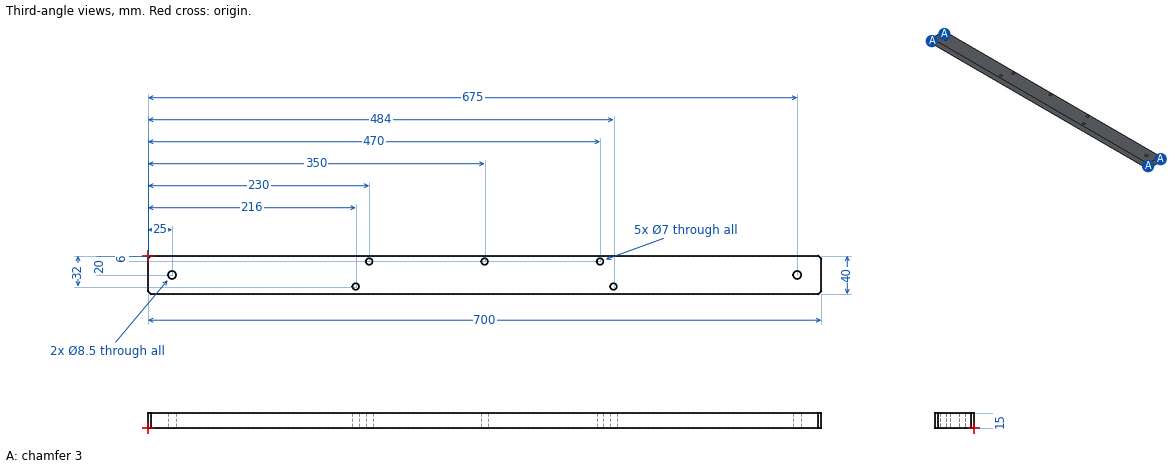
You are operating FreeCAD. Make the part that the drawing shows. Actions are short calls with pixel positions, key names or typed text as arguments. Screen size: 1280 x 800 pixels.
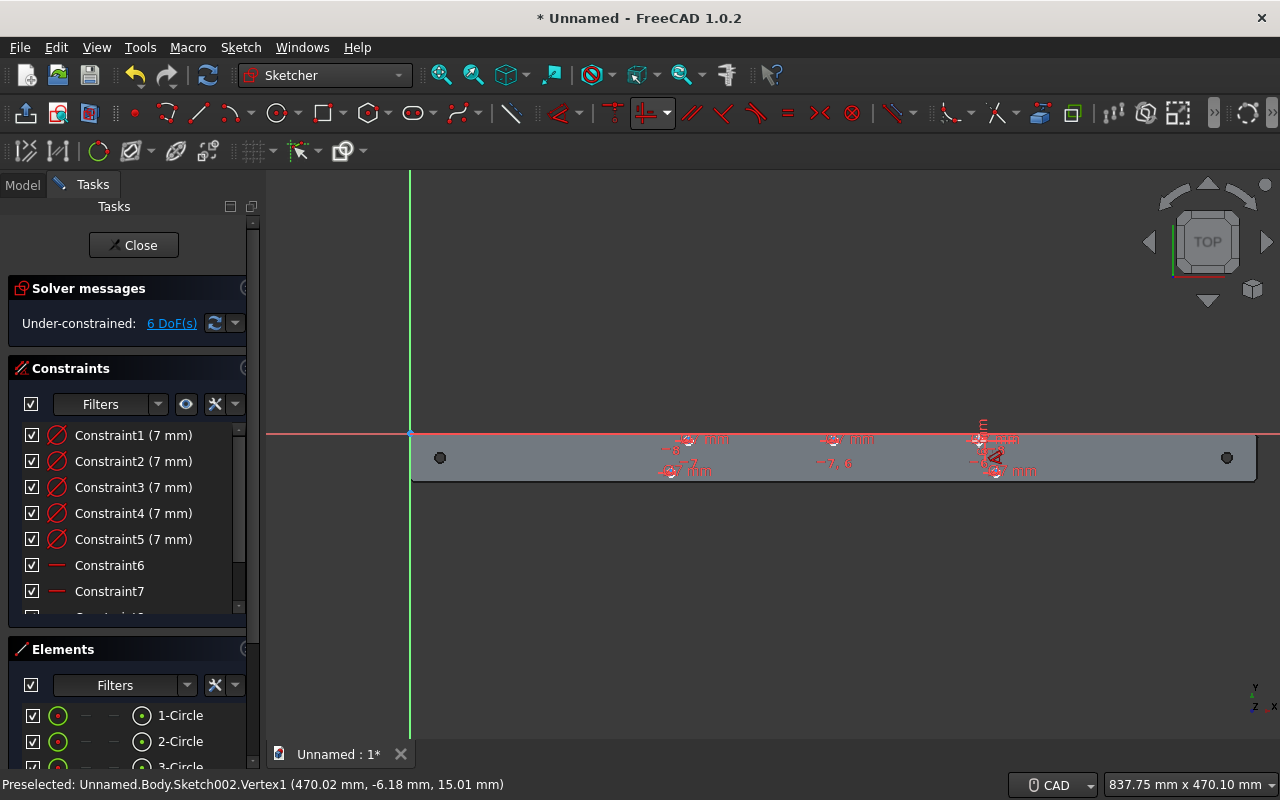
click(671, 473)
click(376, 453)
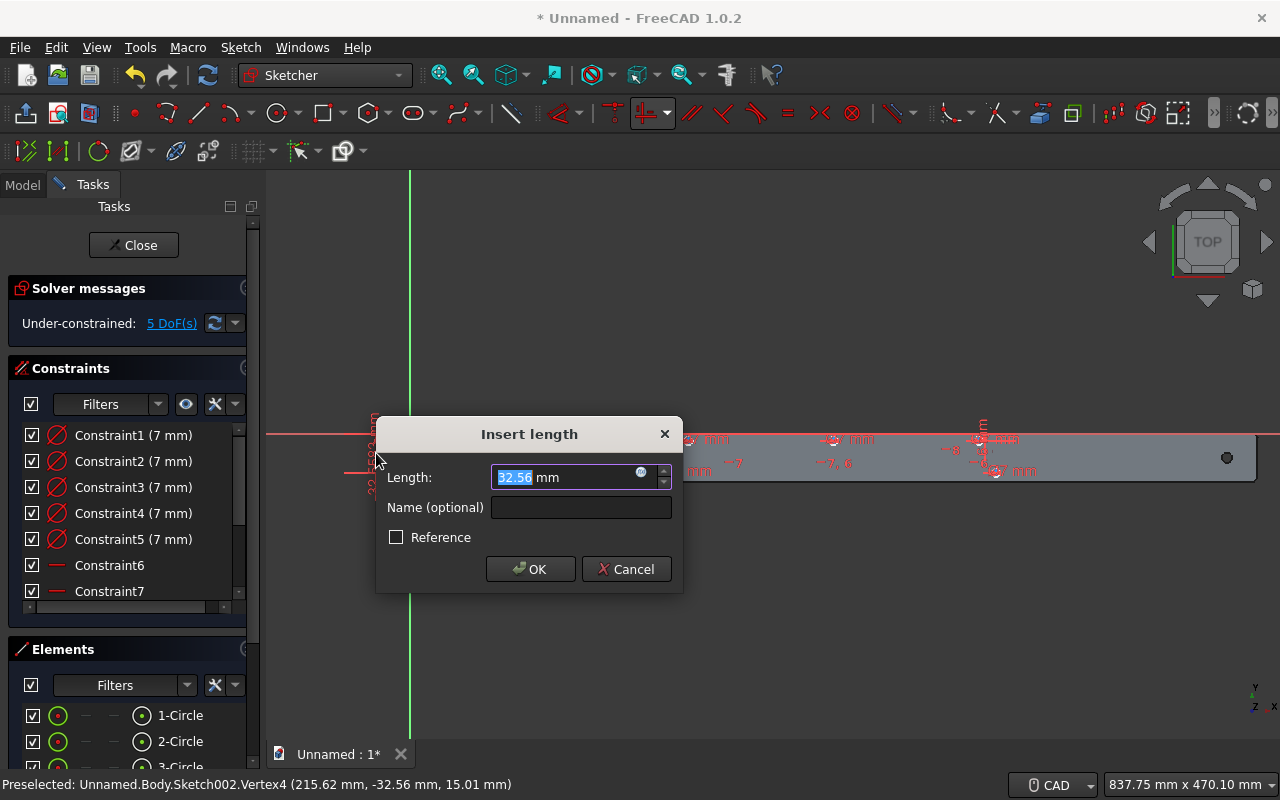
text(32)
key(Return)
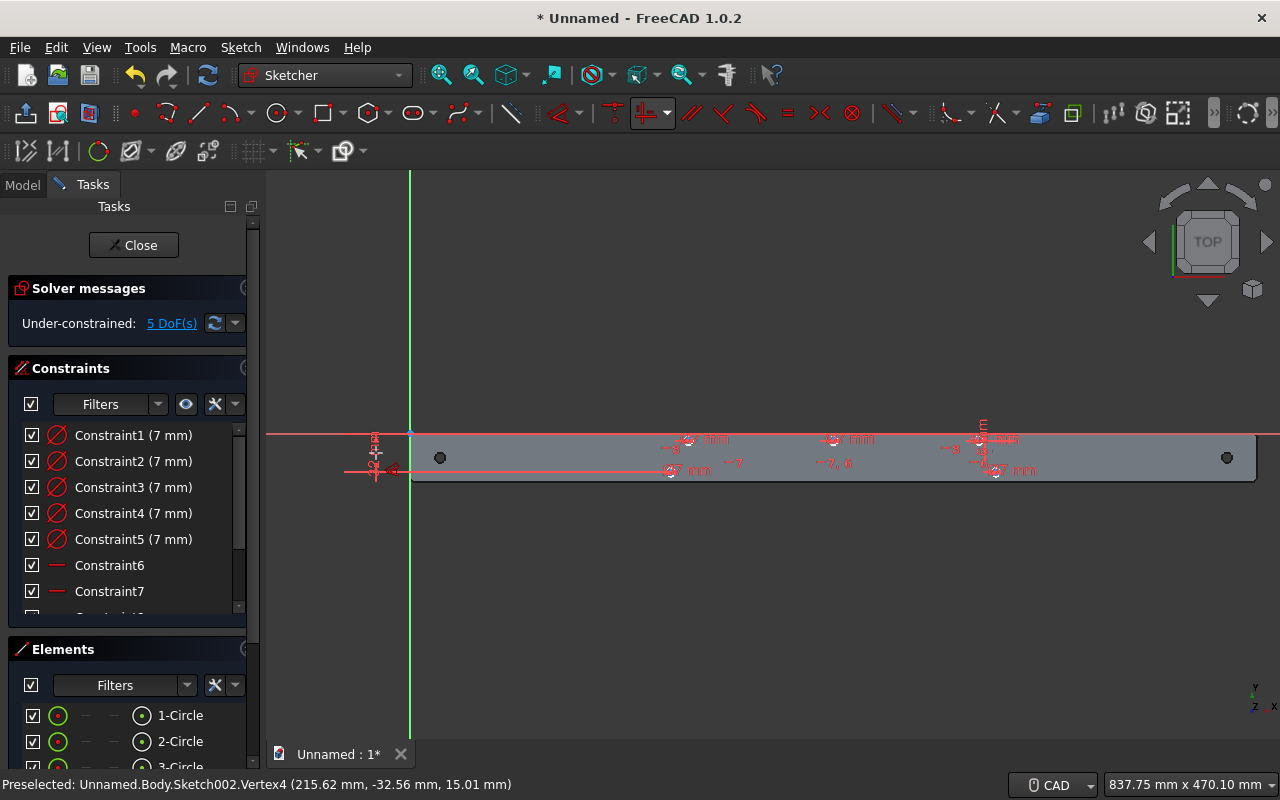
click(979, 441)
click(694, 400)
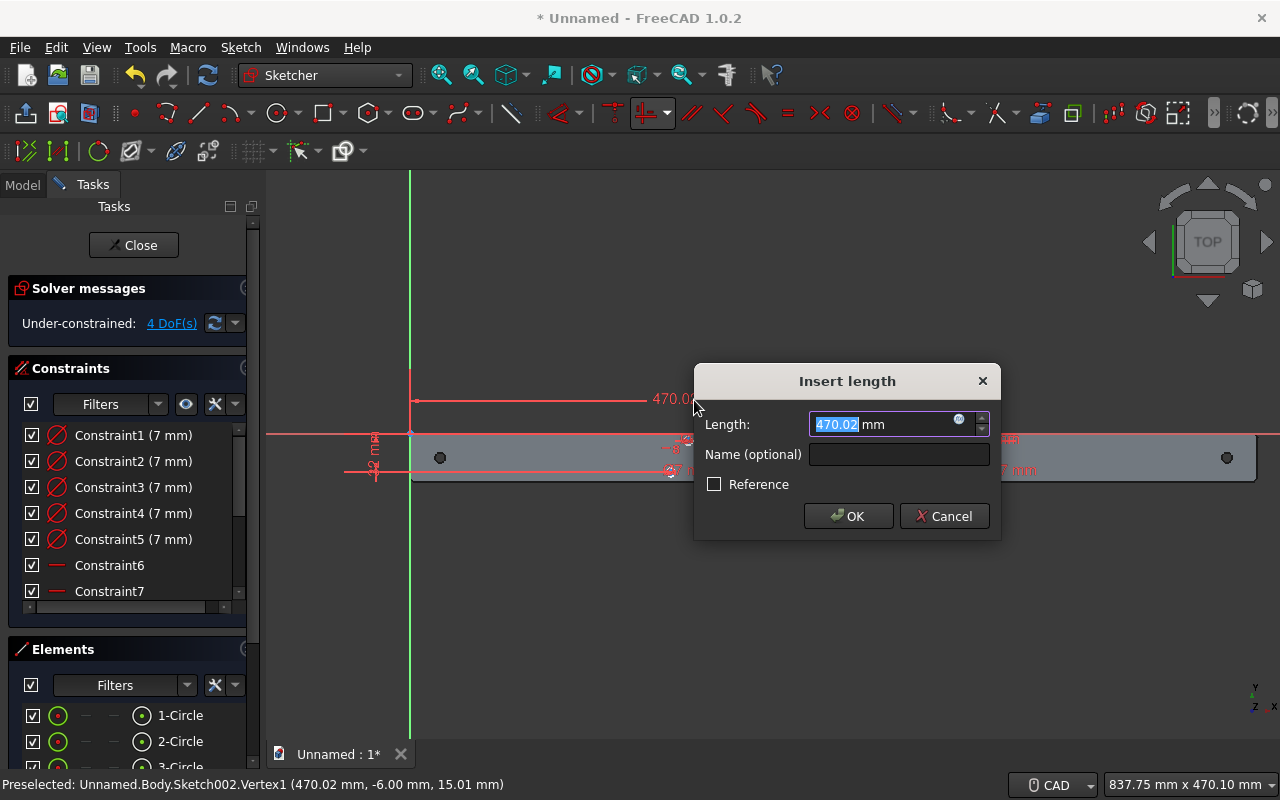
text(470)
key(Return)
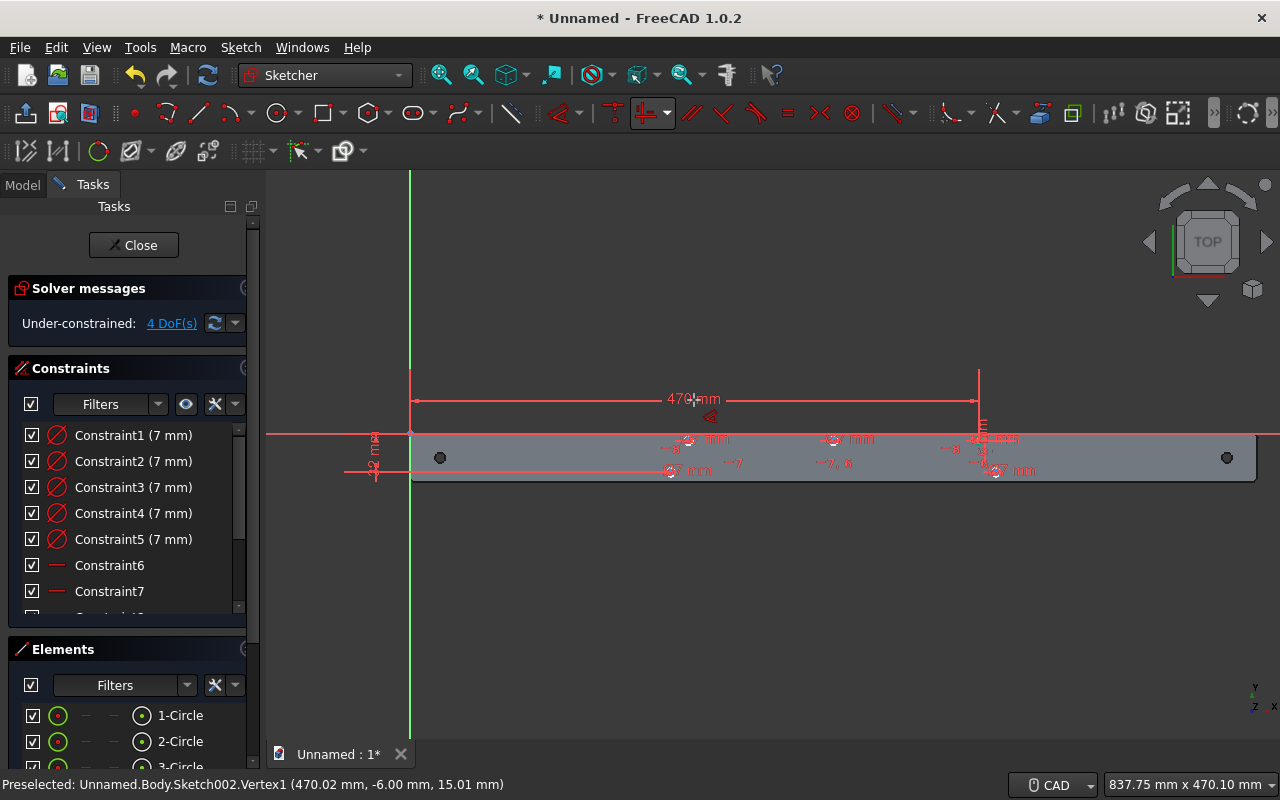
click(834, 441)
click(622, 400)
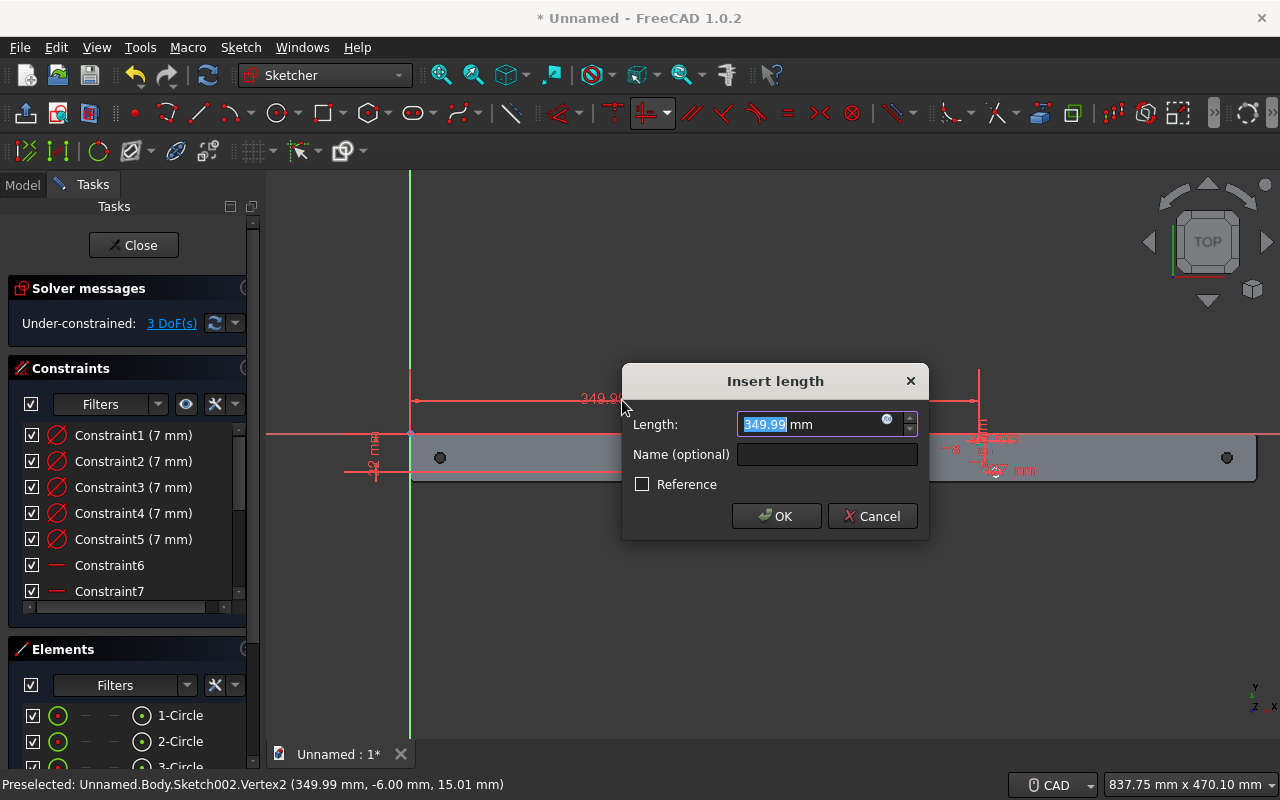
text(350)
key(Return)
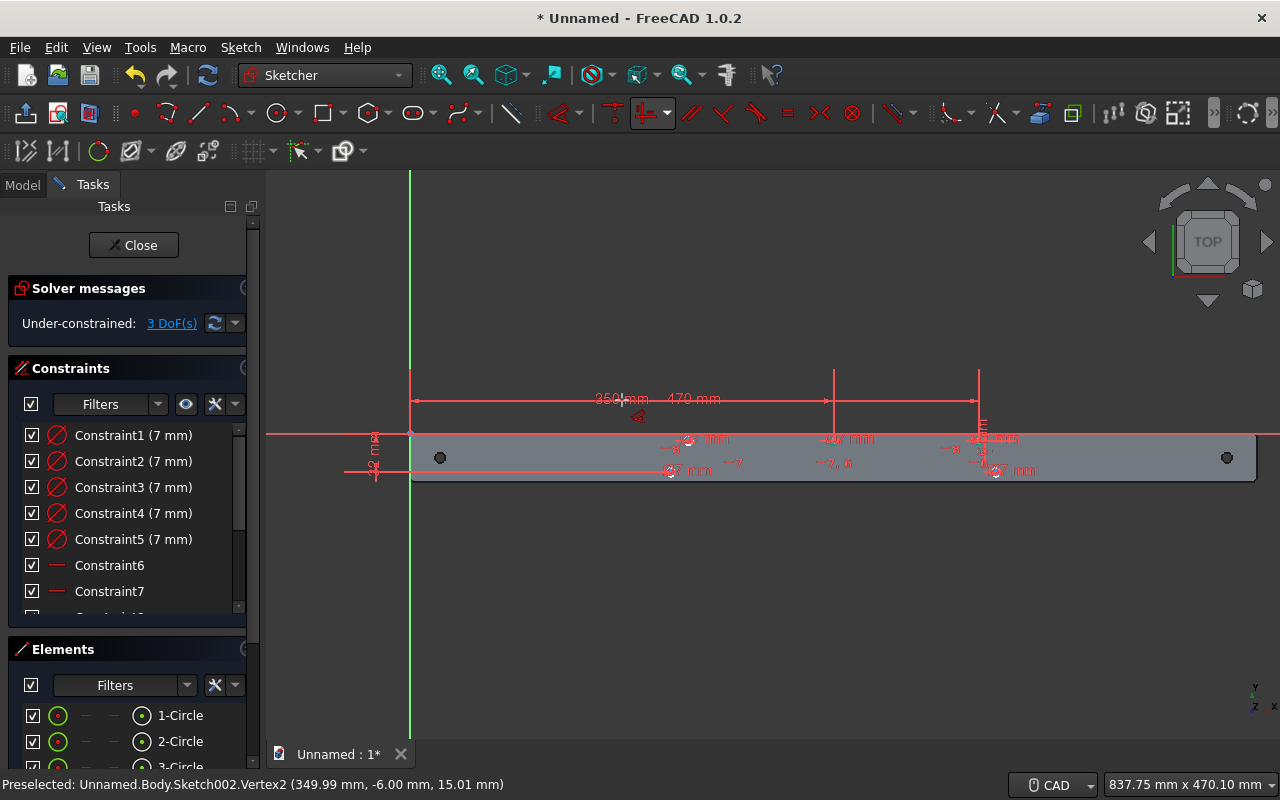
click(688, 441)
click(549, 400)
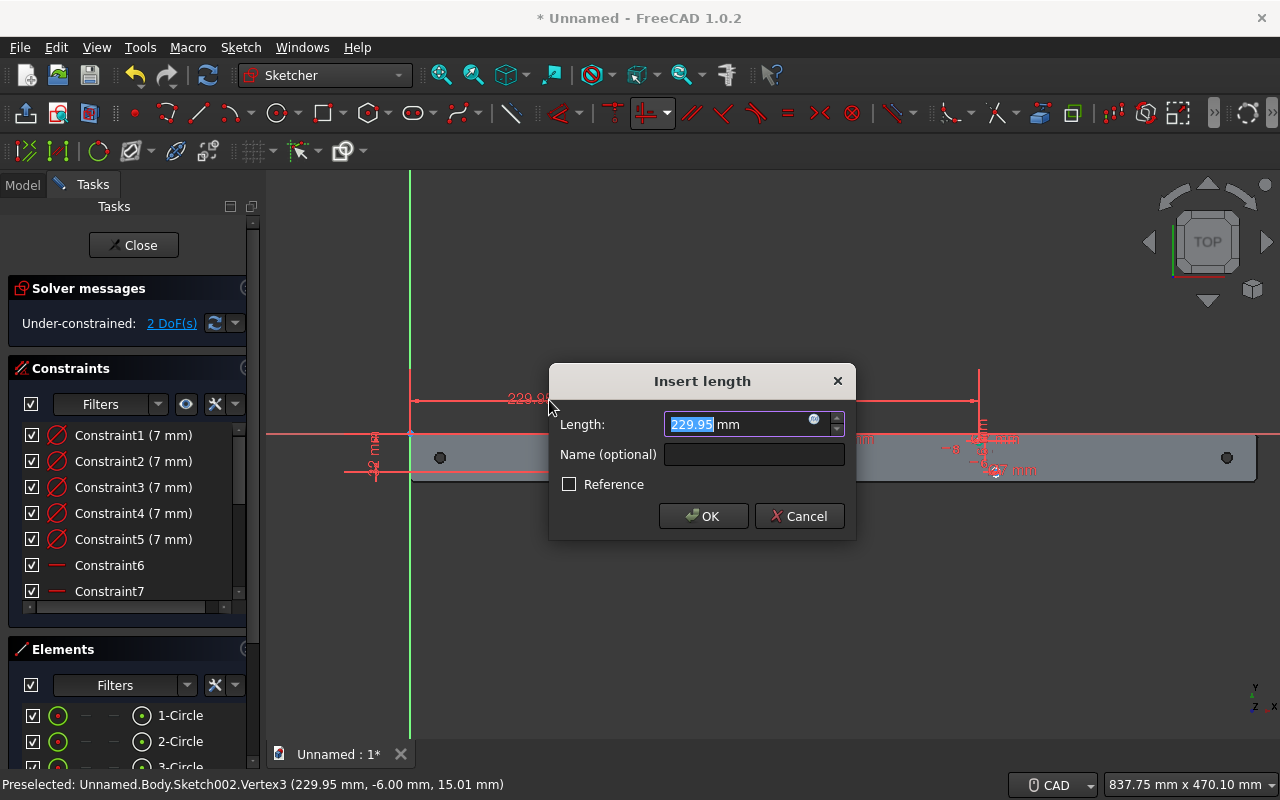
text(230)
key(Return)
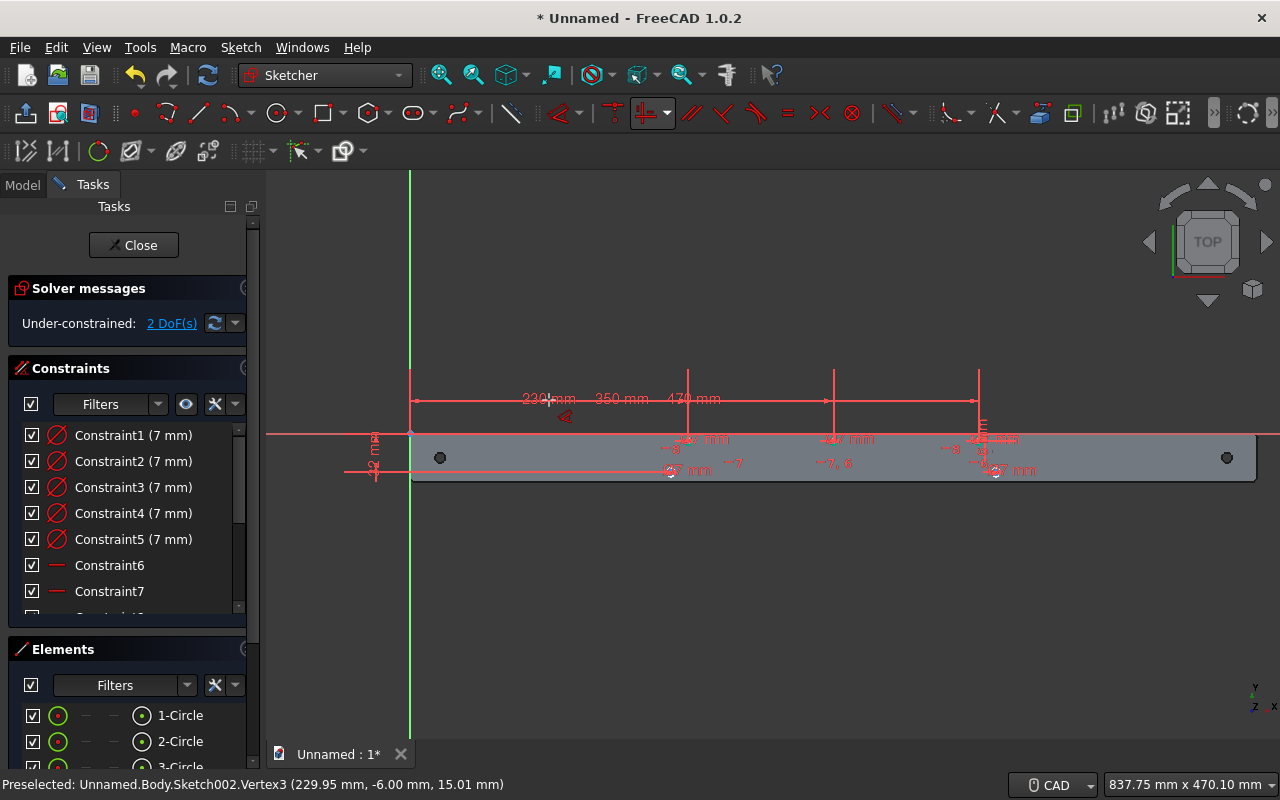
click(671, 472)
click(449, 400)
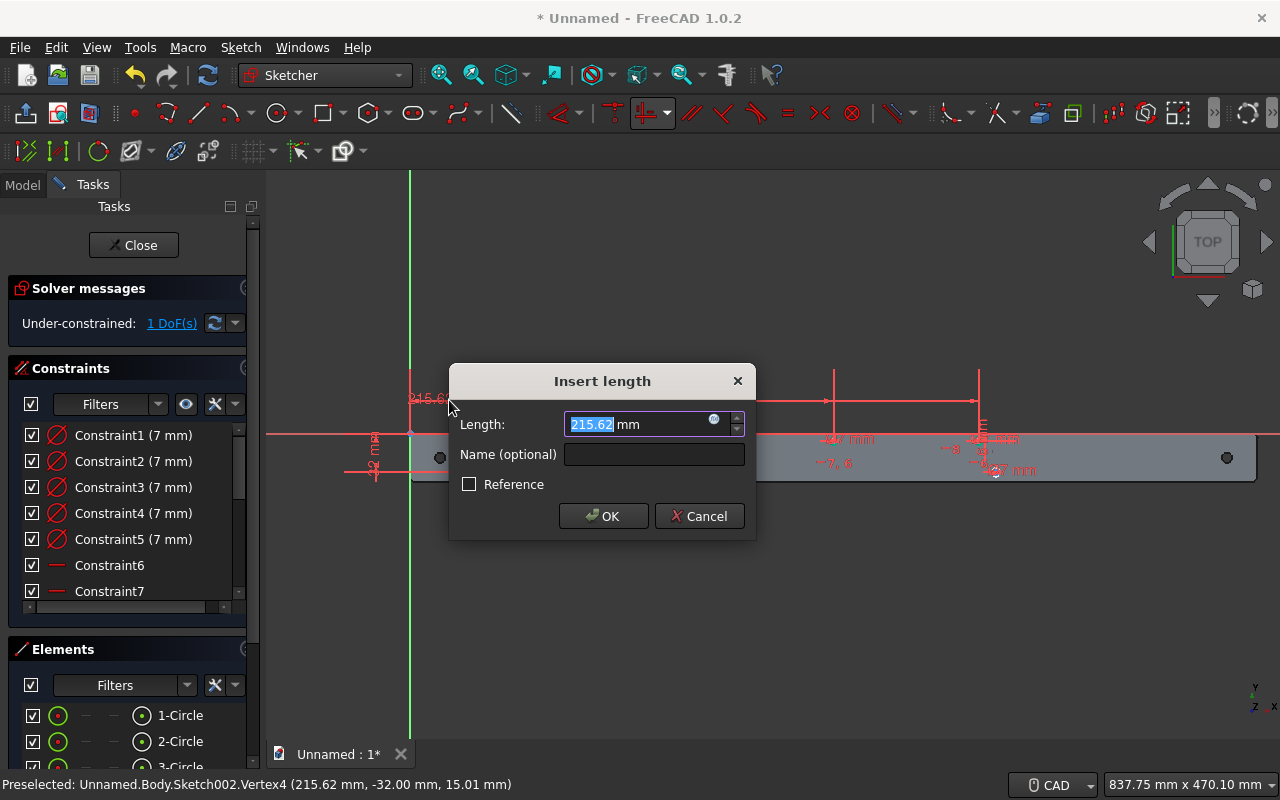
text(216)
key(Return)